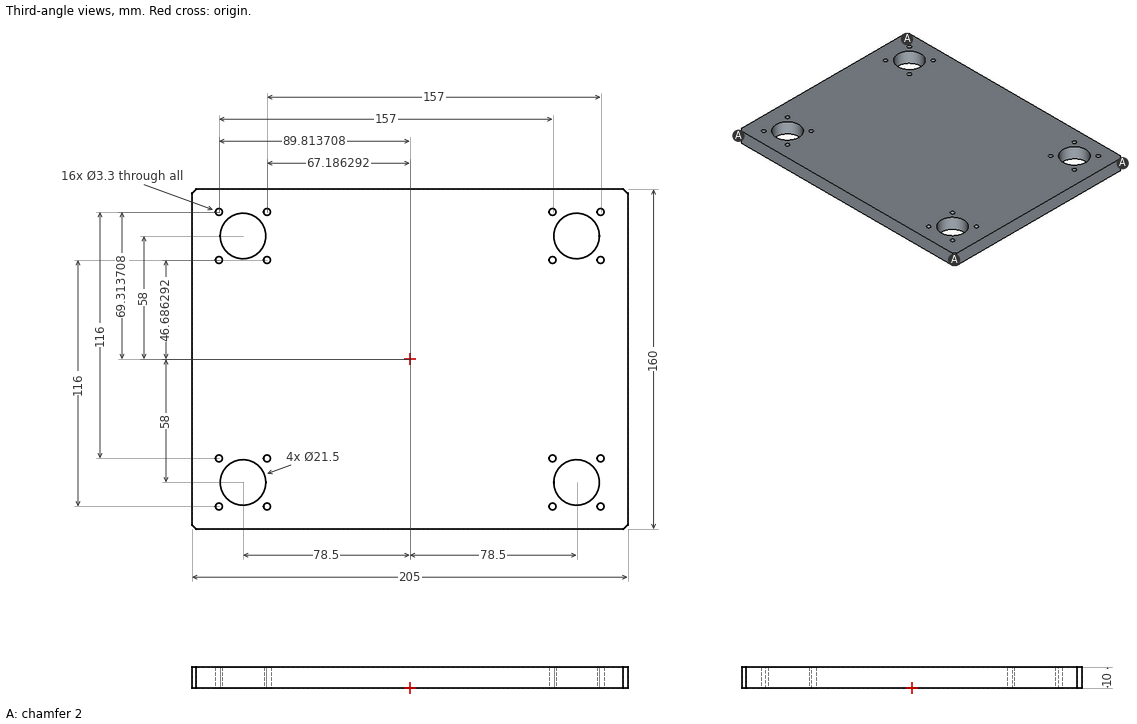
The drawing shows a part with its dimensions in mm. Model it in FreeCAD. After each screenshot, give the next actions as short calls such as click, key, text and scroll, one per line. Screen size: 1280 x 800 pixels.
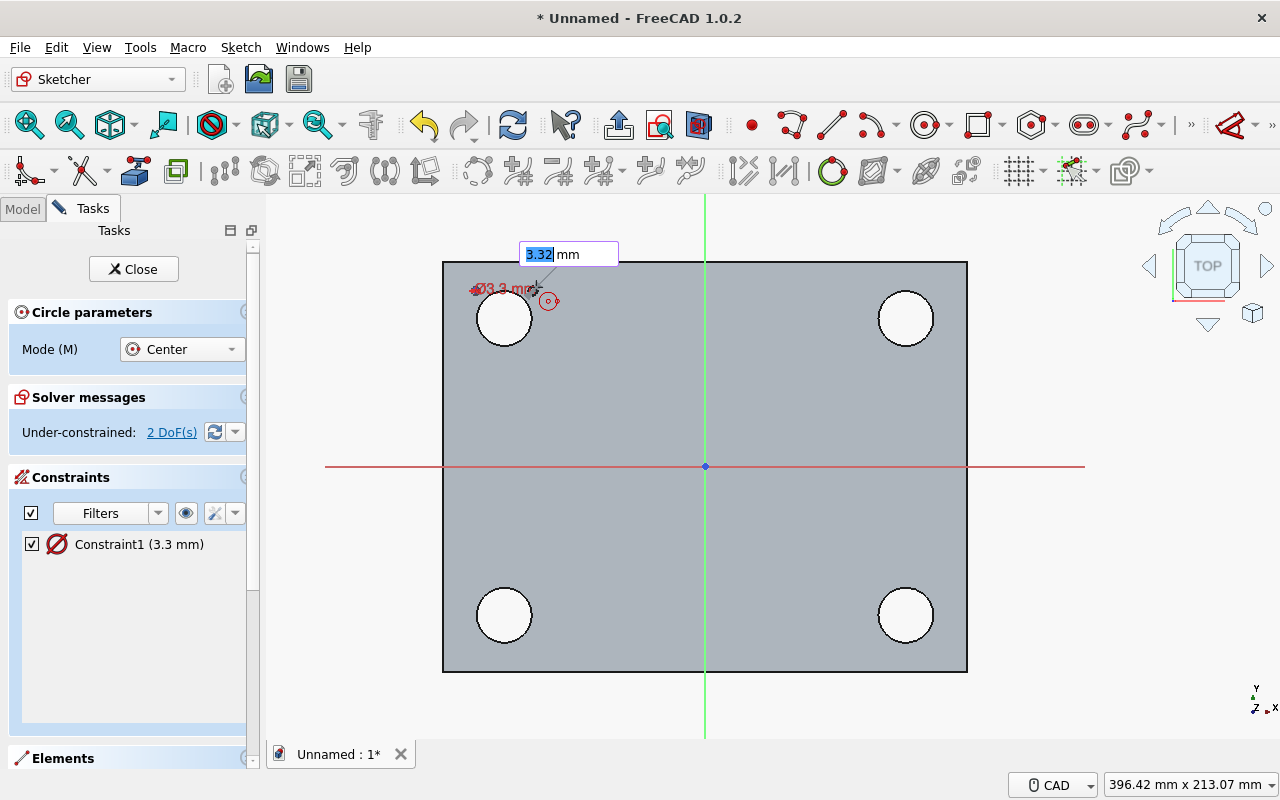
text(3.3)
key(Return)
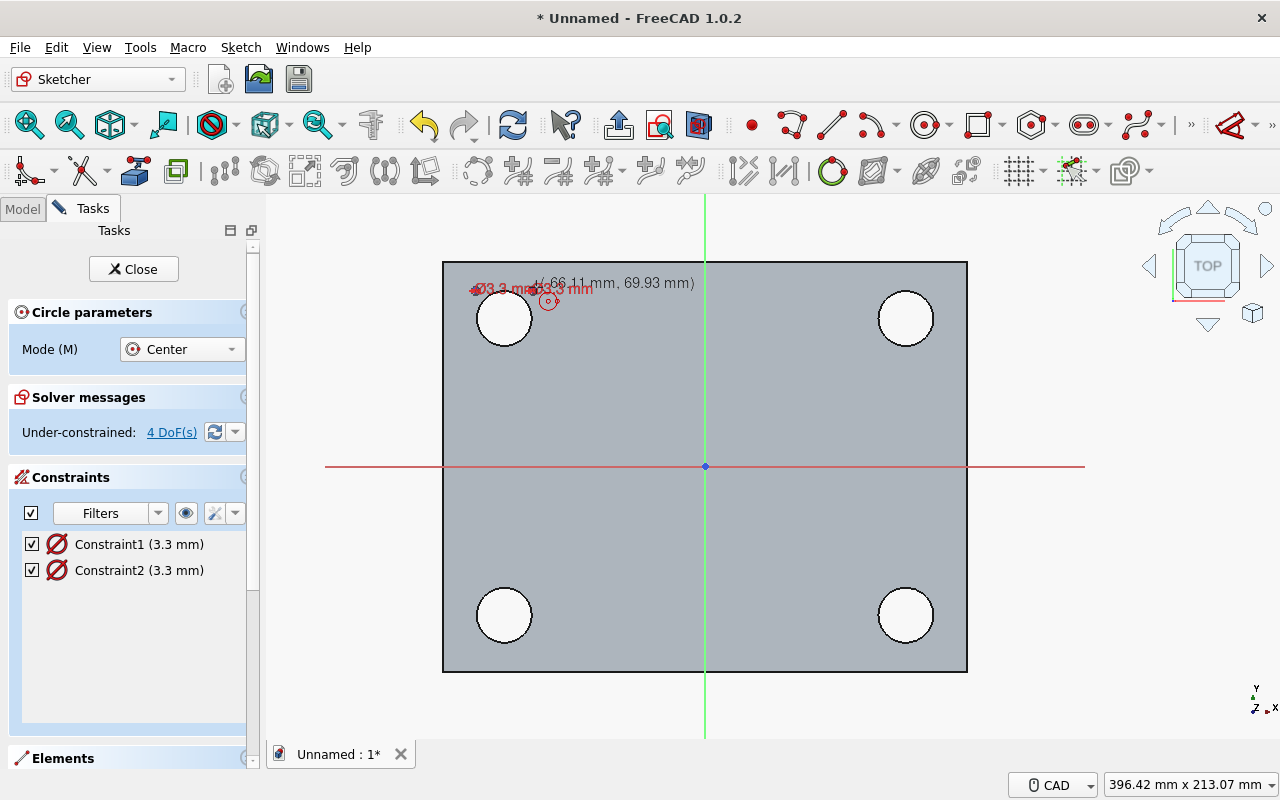
scroll(533, 347, up, 9)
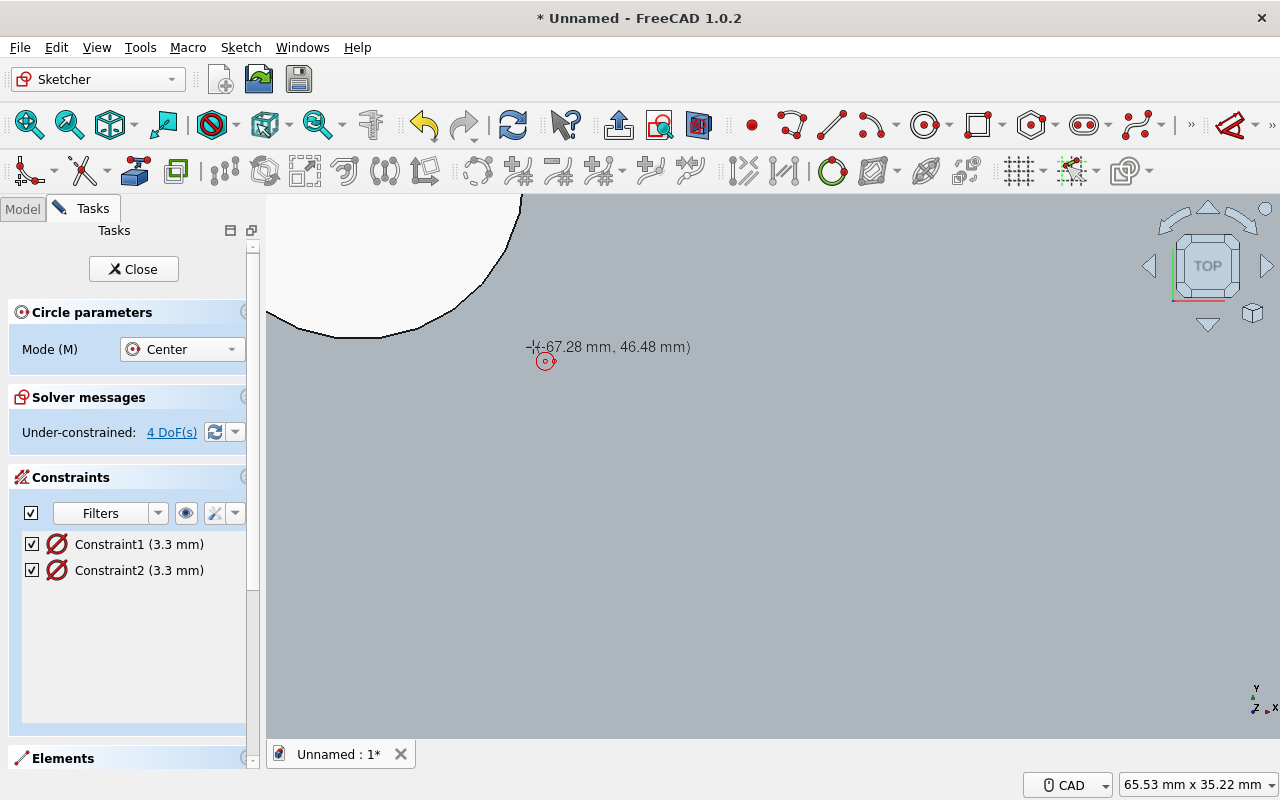
scroll(533, 347, down, 9)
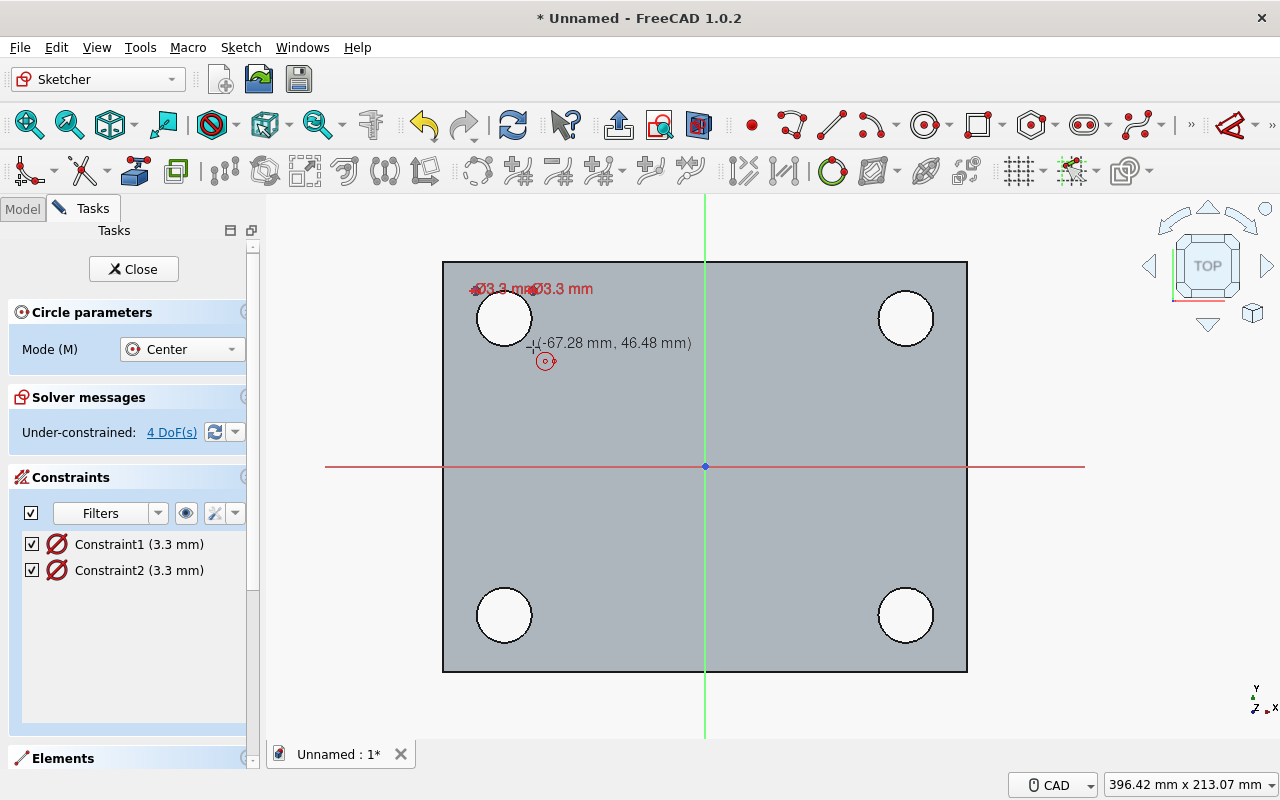
click(533, 347)
move(536, 344)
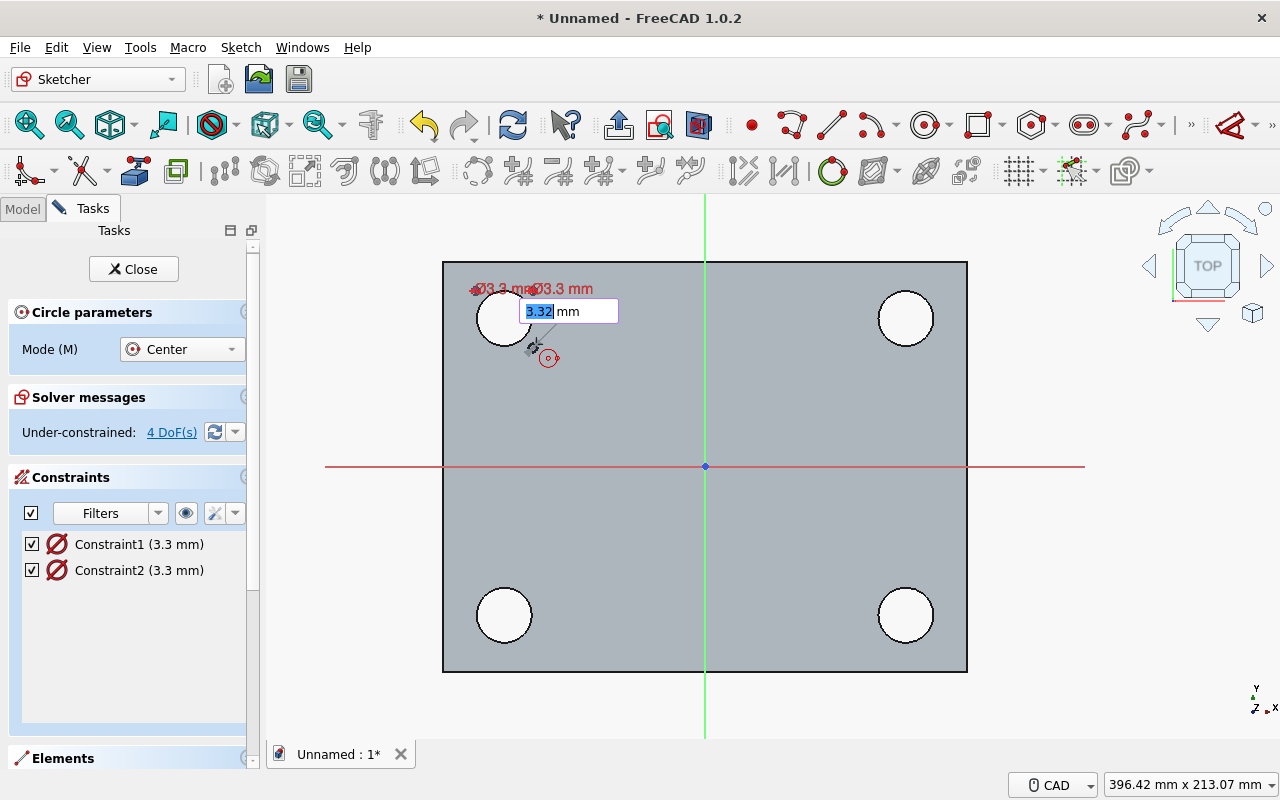
text(3.3)
key(Return)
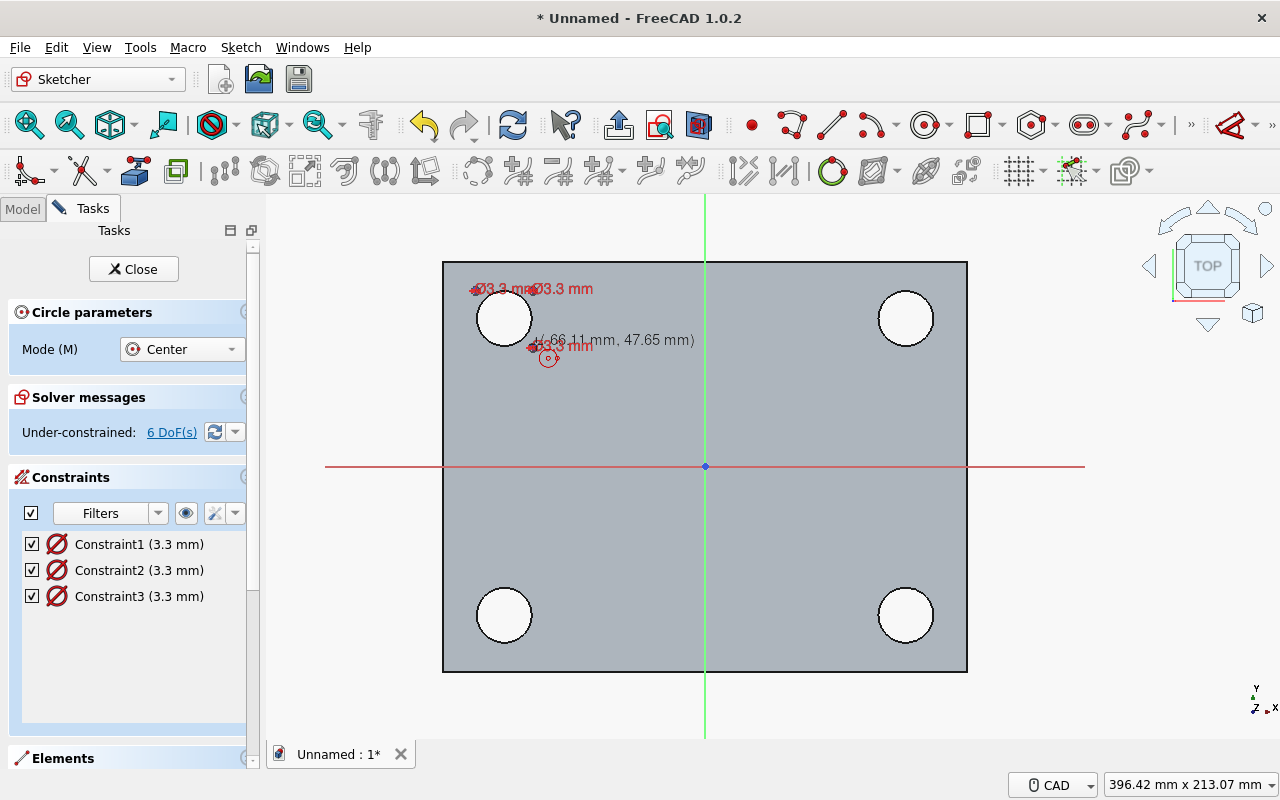
scroll(475, 347, up, 9)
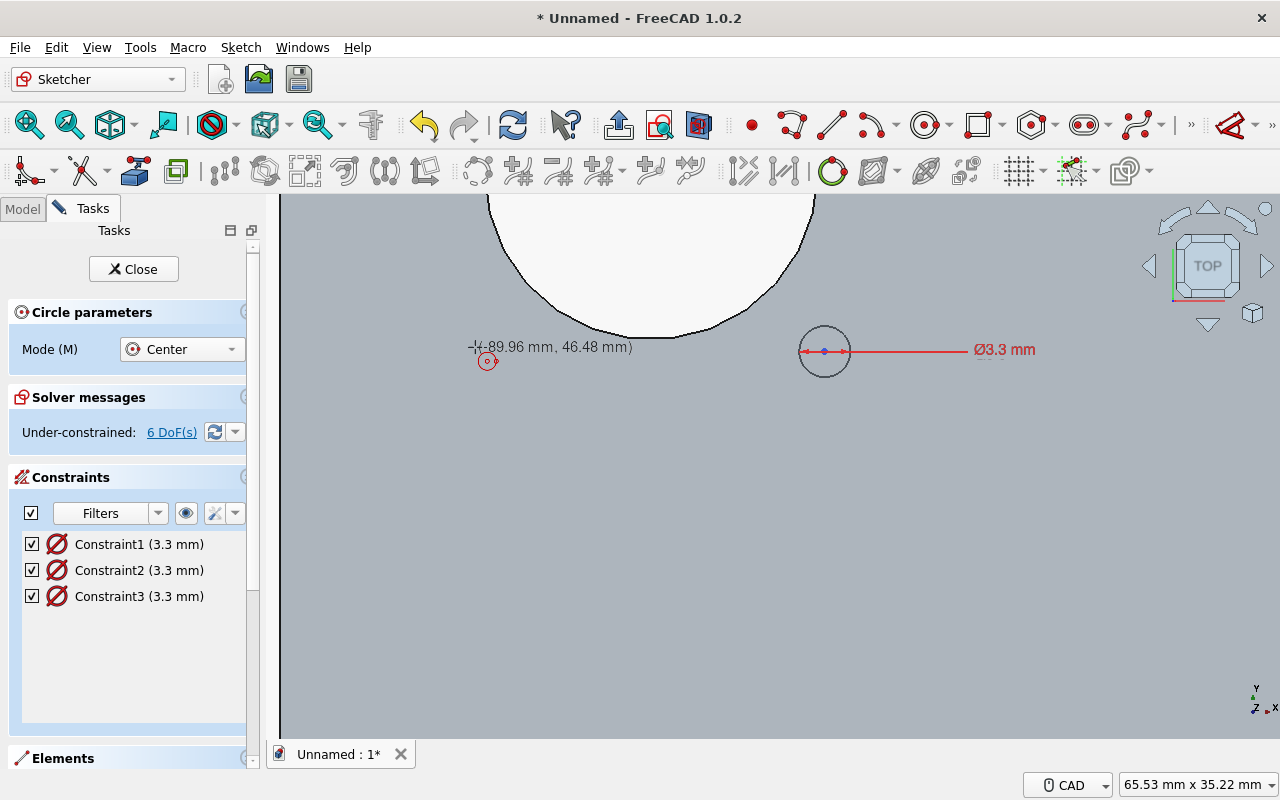
scroll(474, 347, down, 9)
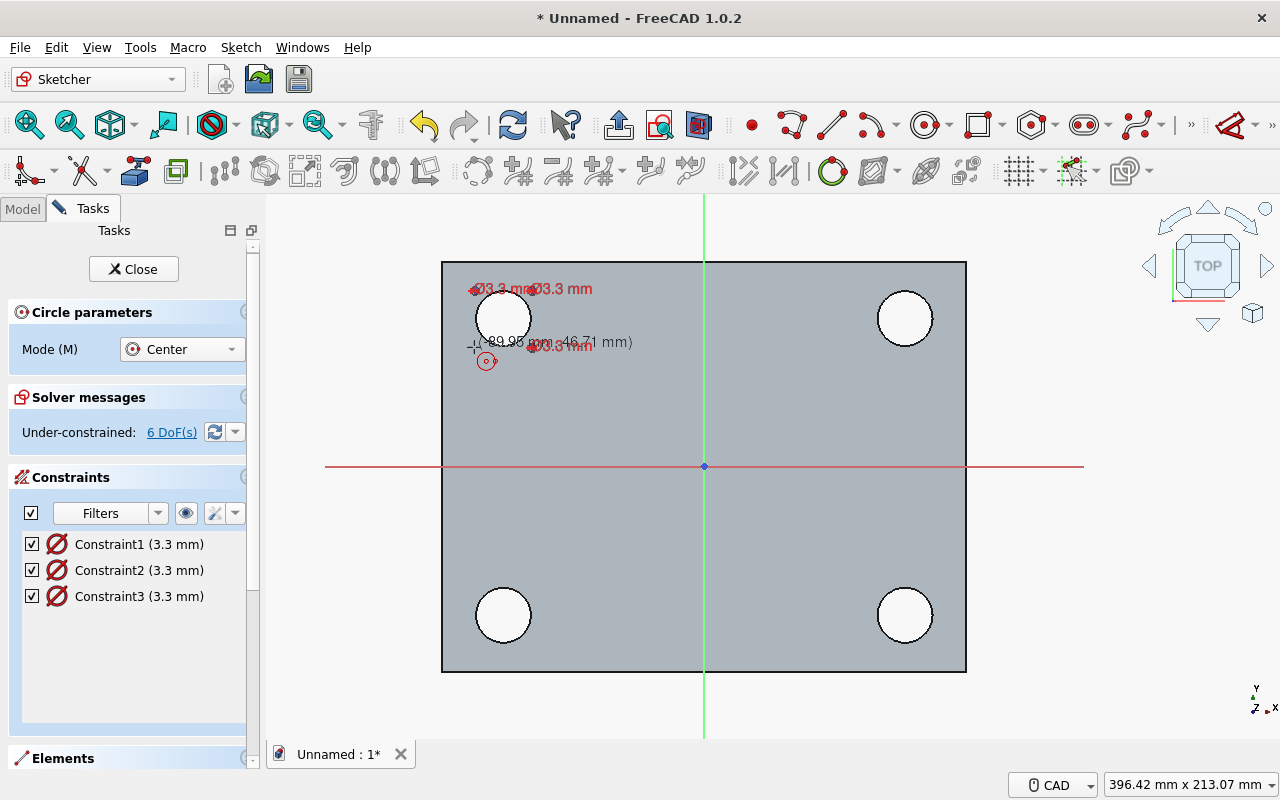
click(475, 347)
move(478, 344)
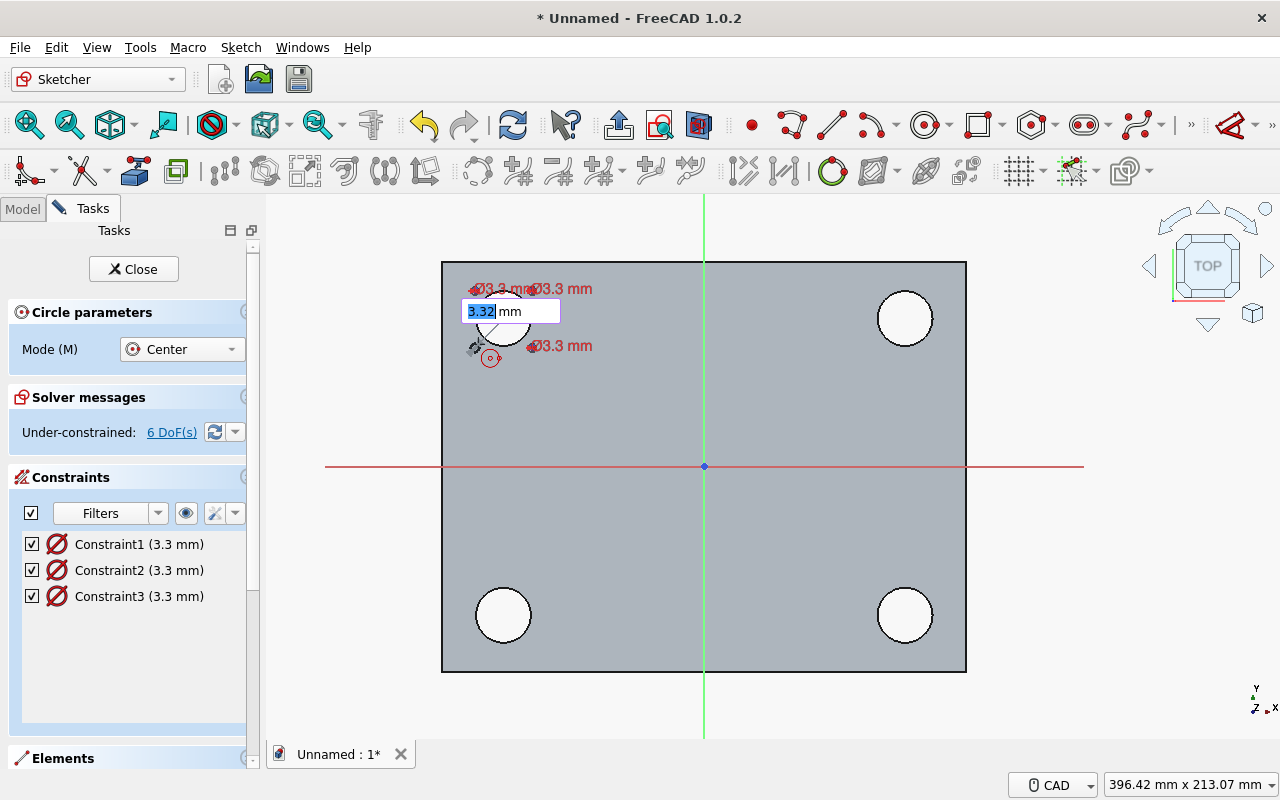
text(3.3)
key(Return)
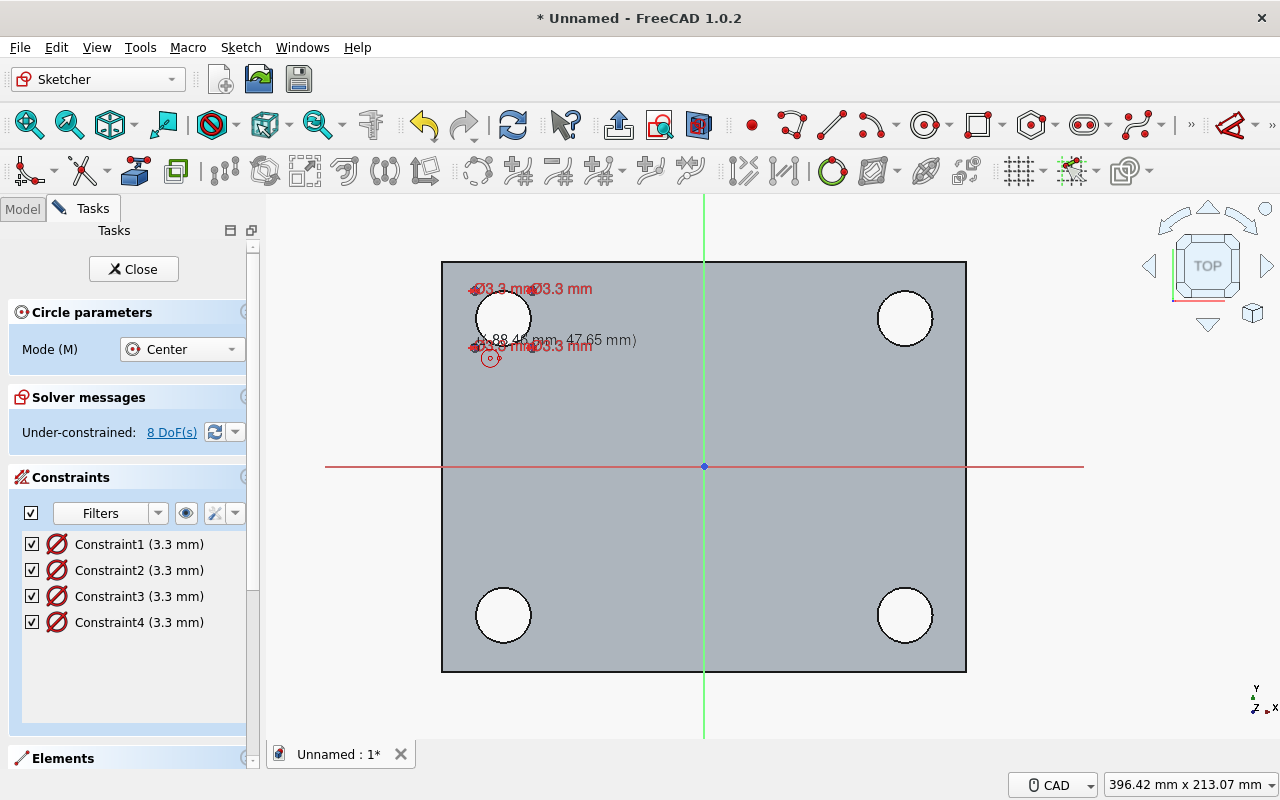
scroll(876, 290, up, 9)